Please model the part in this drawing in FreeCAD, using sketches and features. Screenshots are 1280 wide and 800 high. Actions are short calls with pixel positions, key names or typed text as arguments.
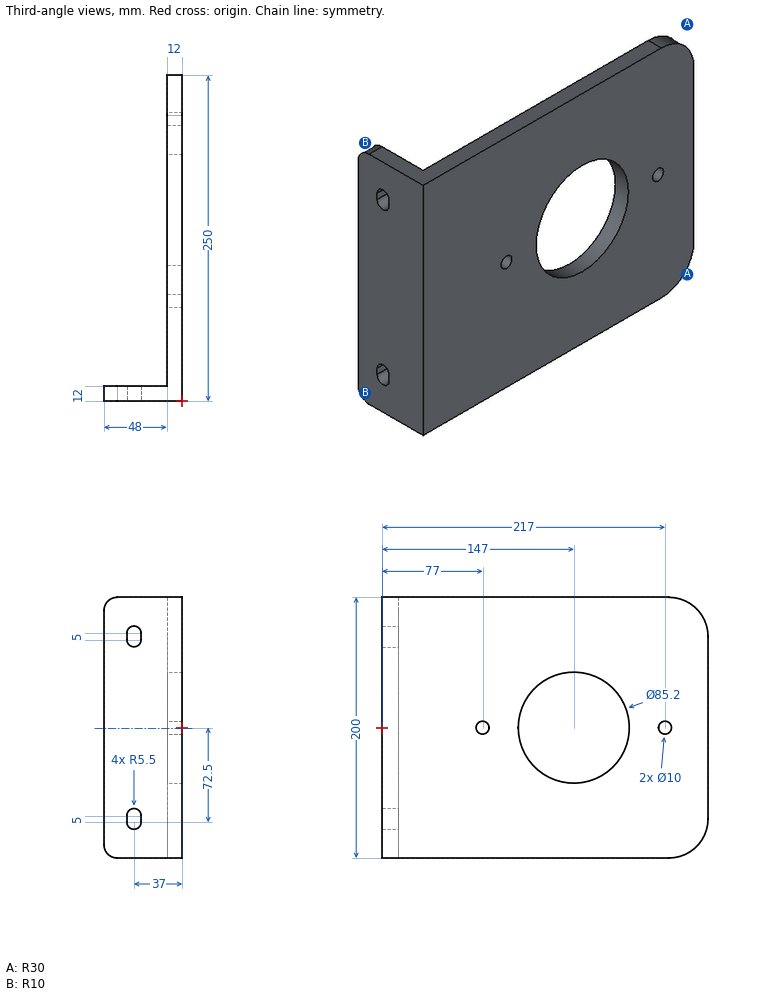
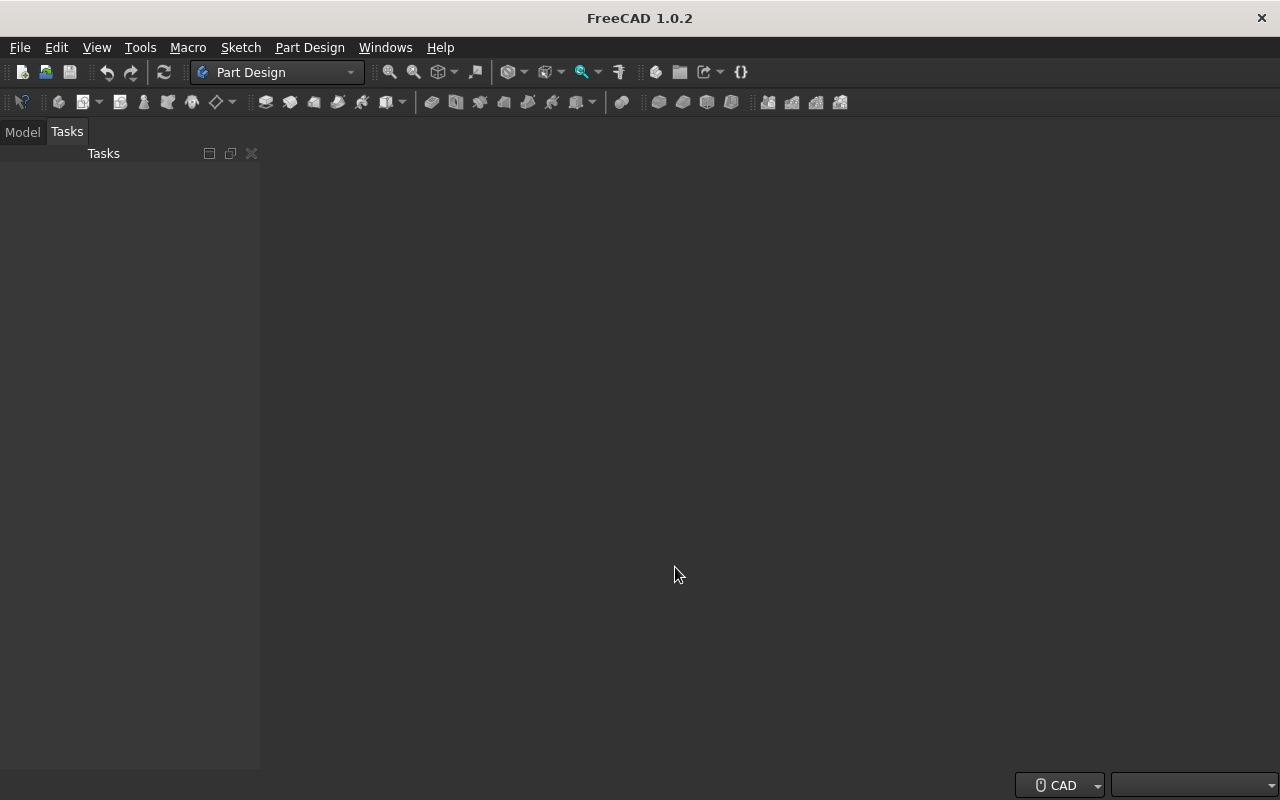
key(ctrl+n)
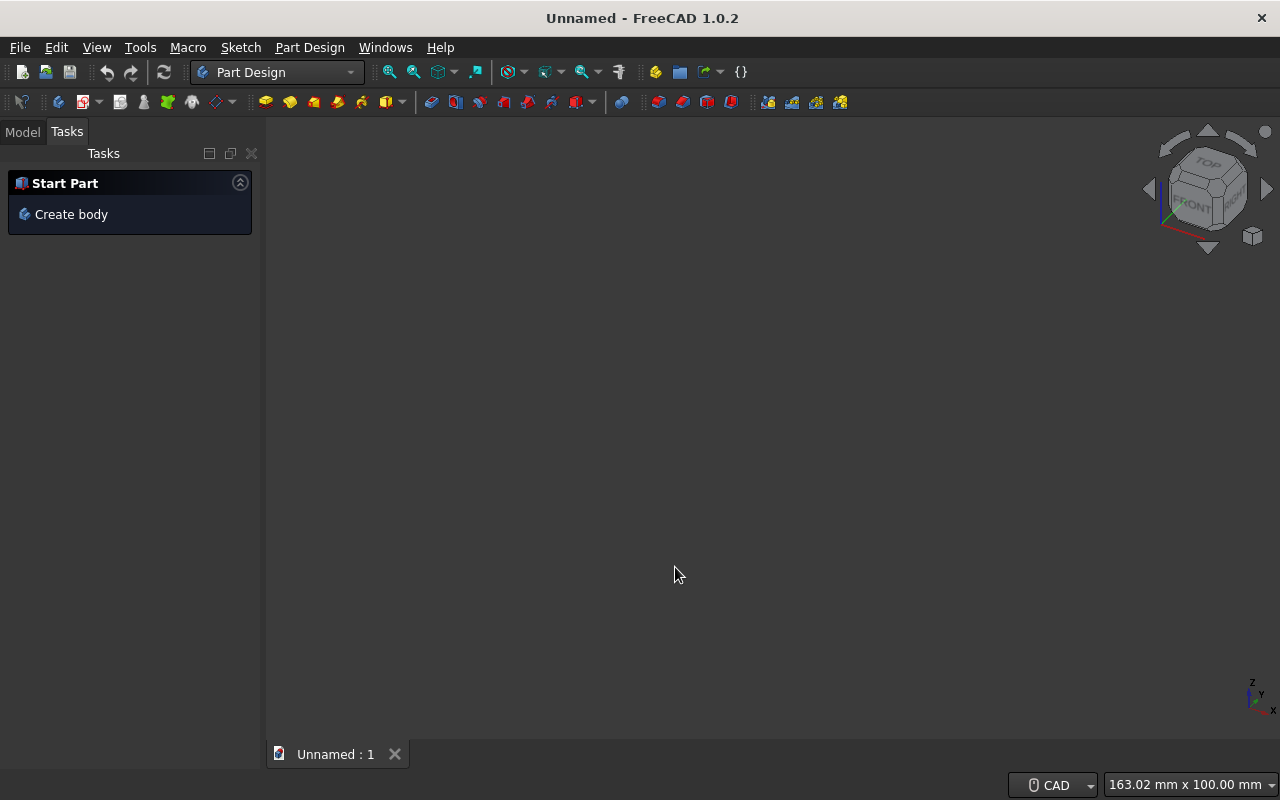
click(84, 102)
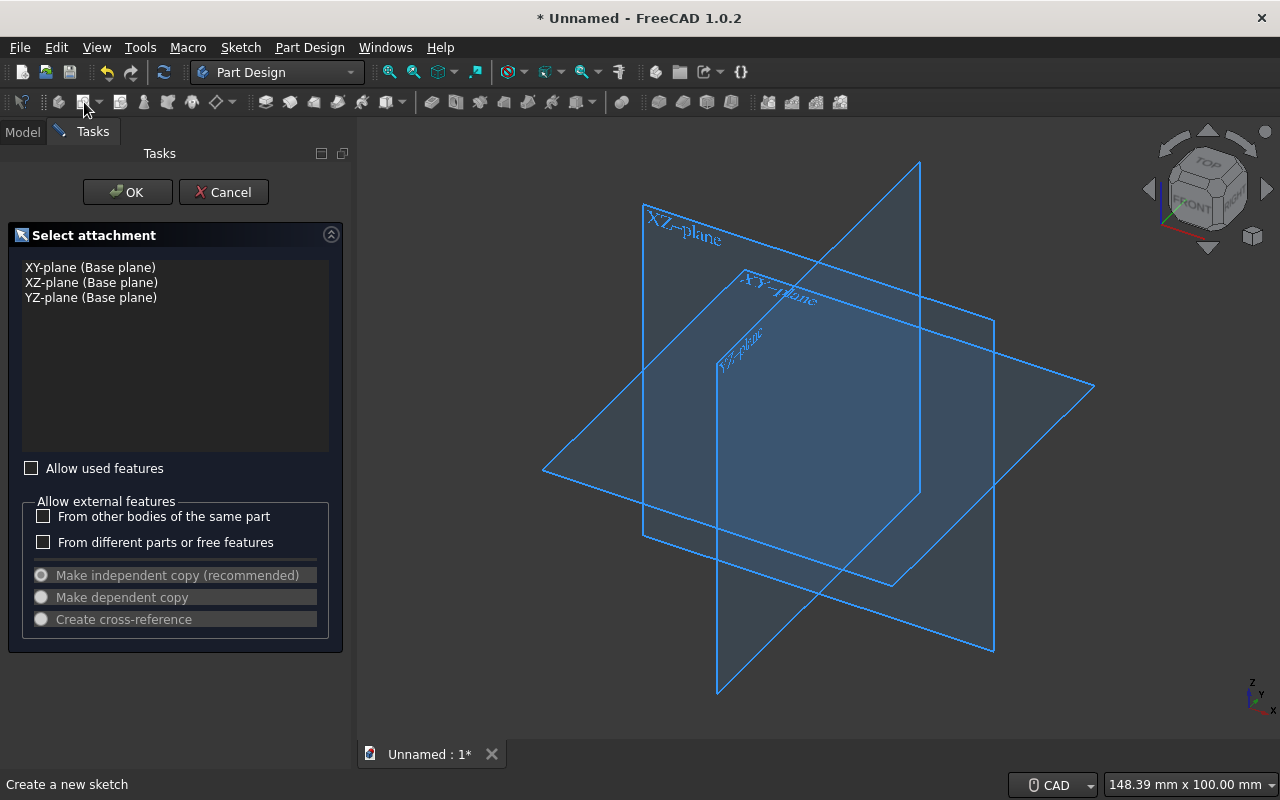
click(82, 268)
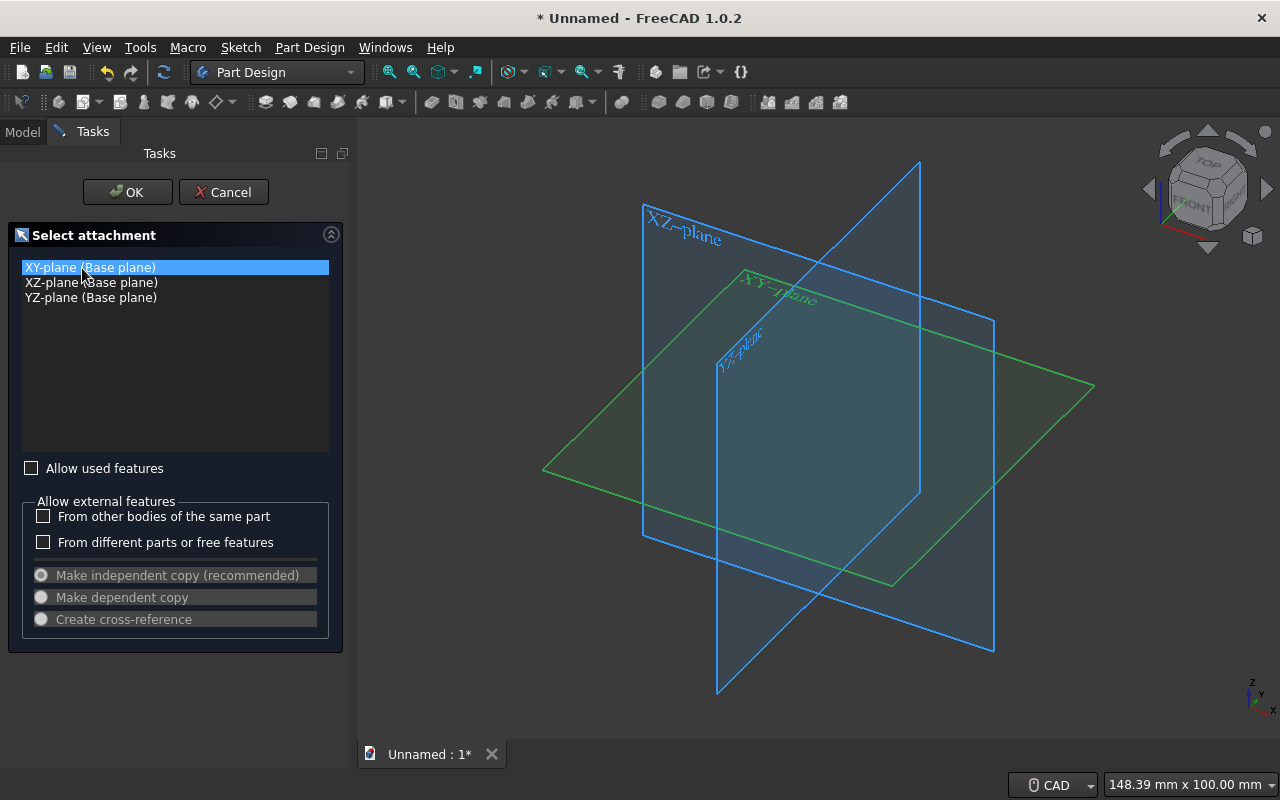
click(128, 192)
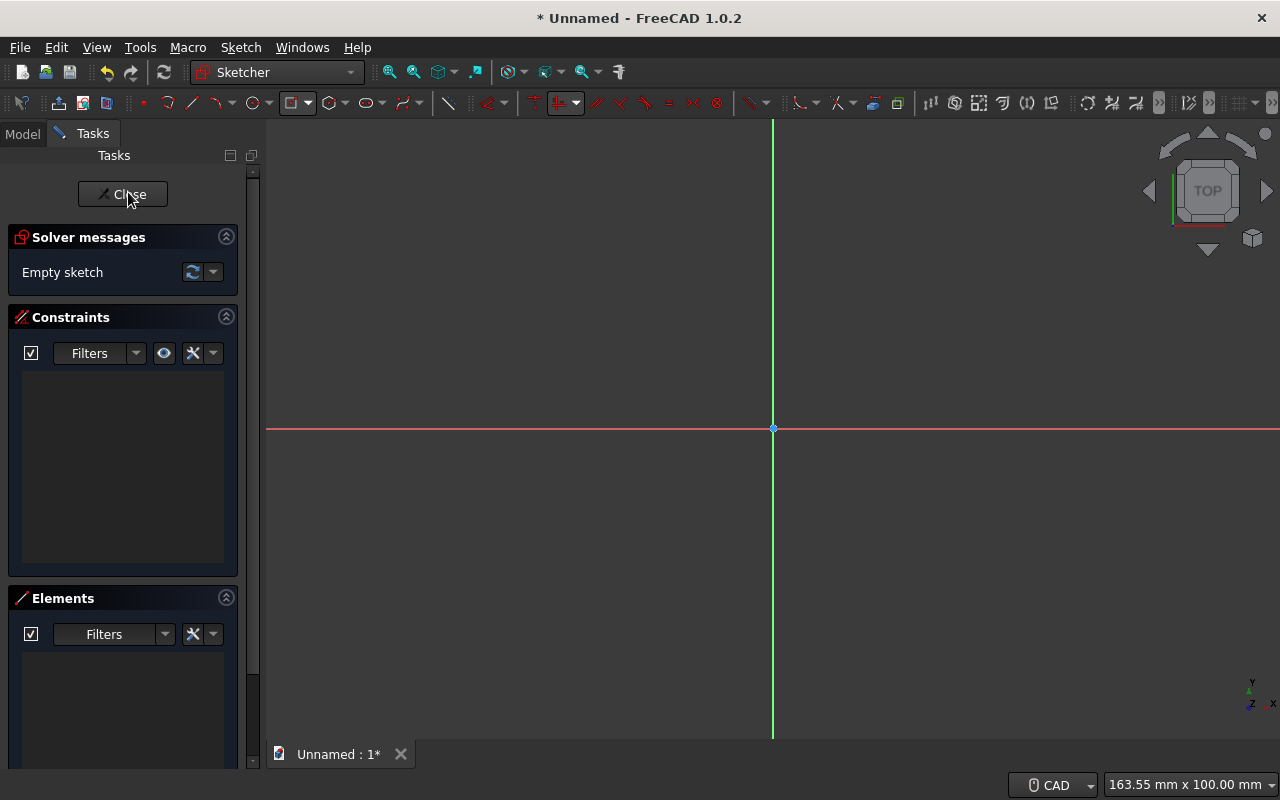
scroll(743, 683, down, 7)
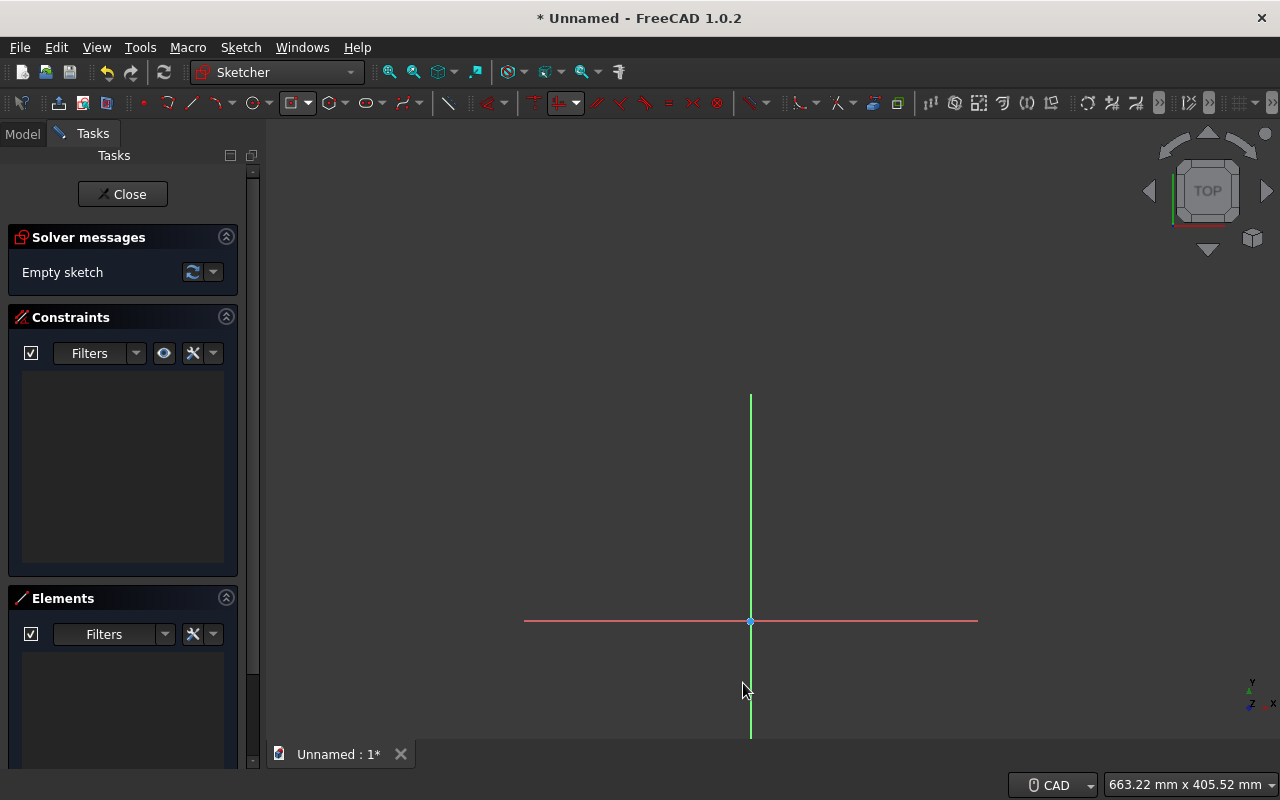
key(g)
key(m)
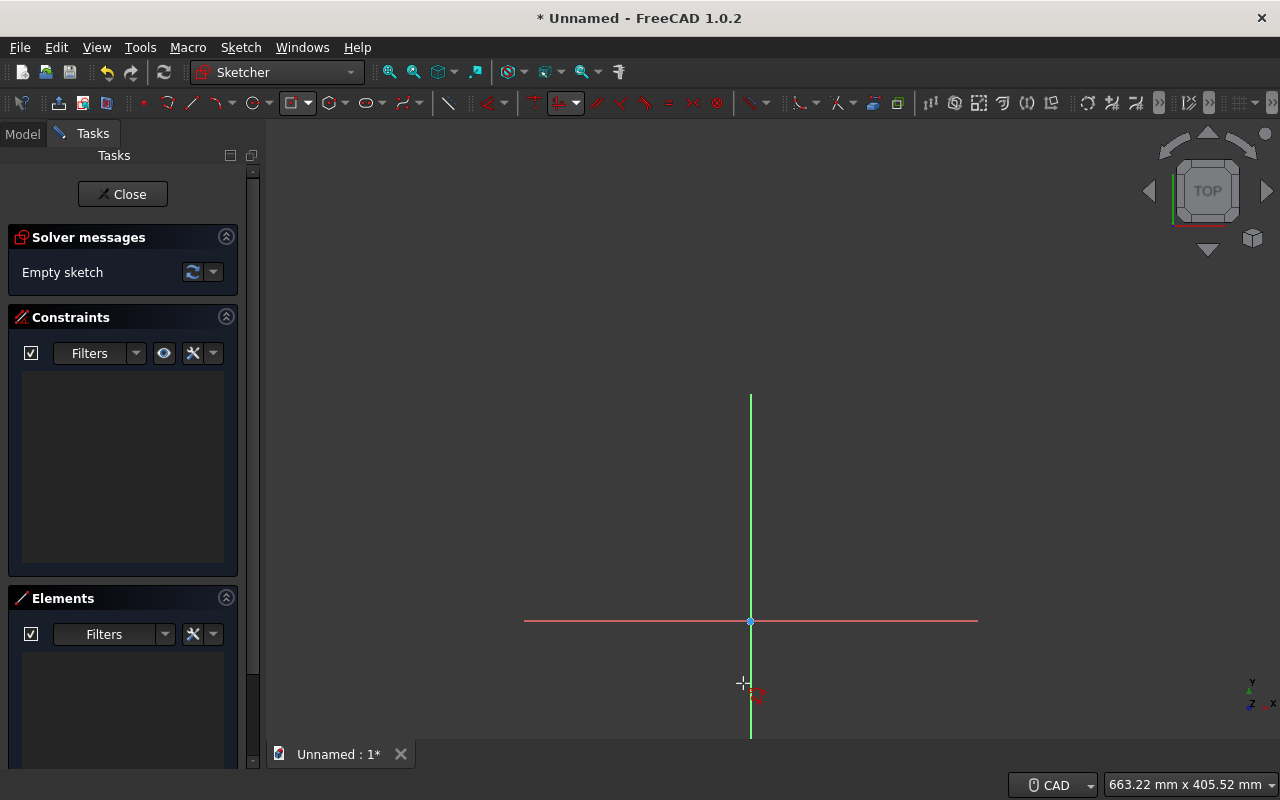
click(751, 621)
click(742, 239)
click(732, 239)
click(732, 603)
click(659, 603)
click(659, 612)
click(751, 621)
key(Escape)
key(Escape)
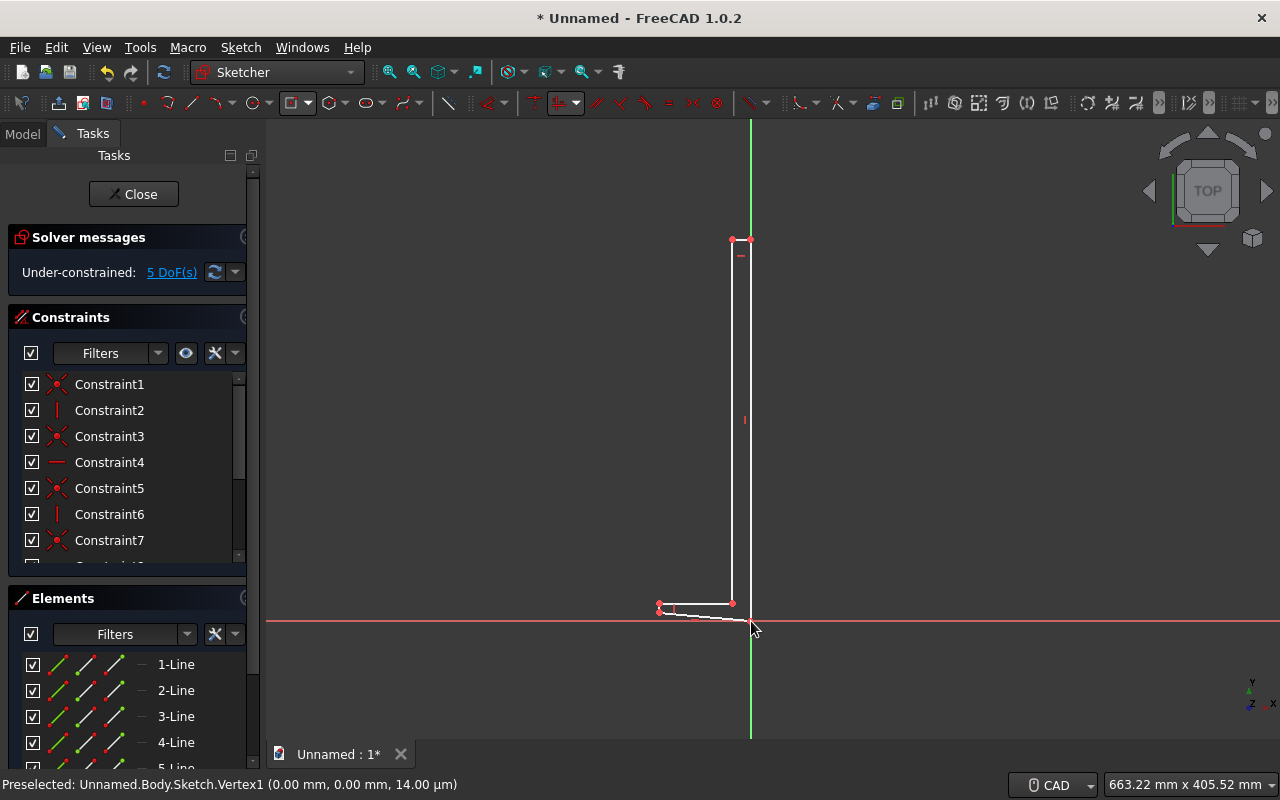
click(723, 619)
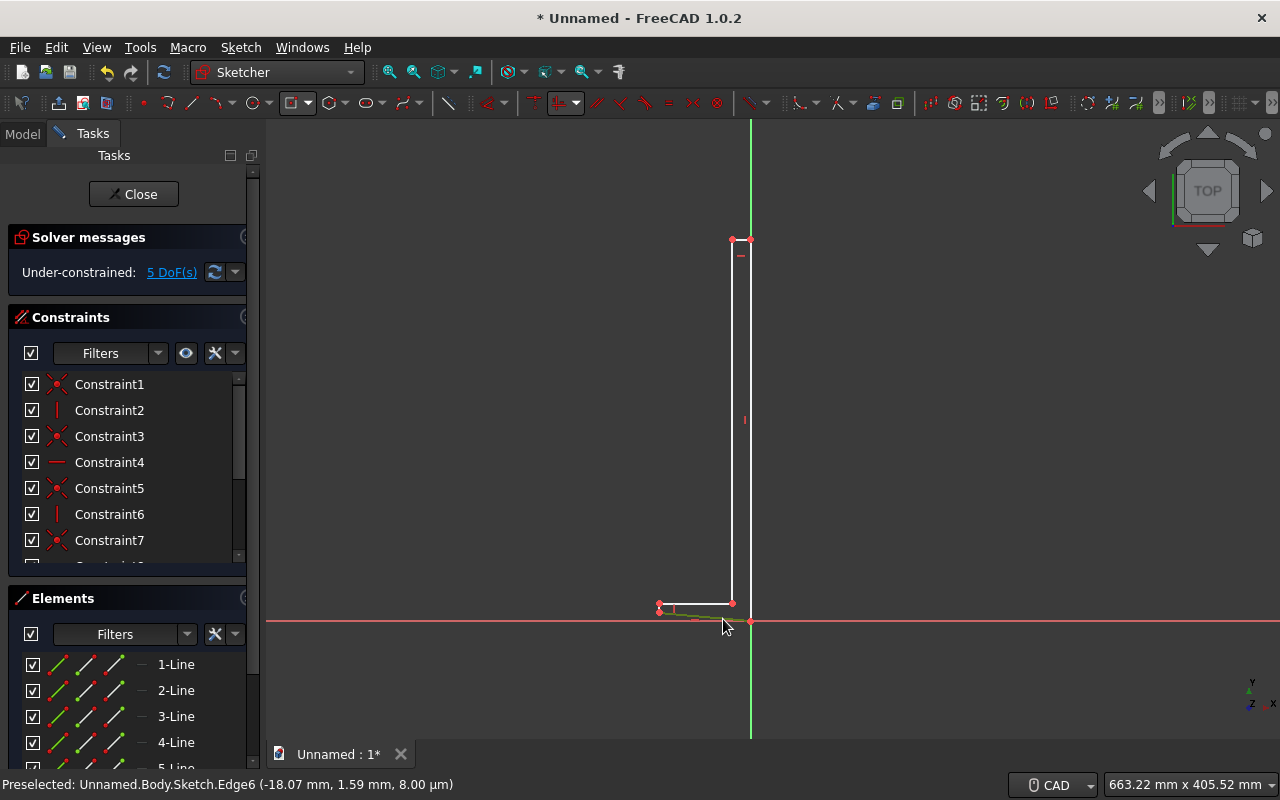
click(578, 104)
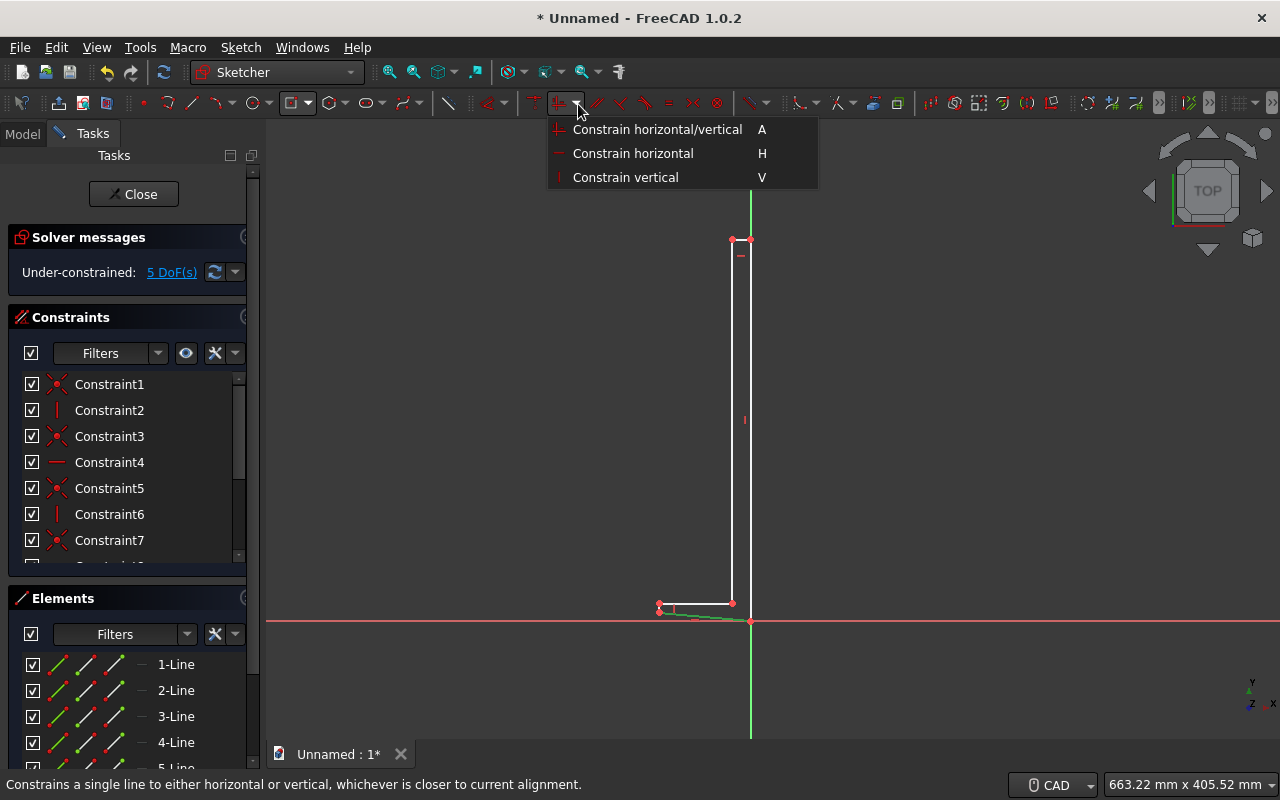
click(683, 153)